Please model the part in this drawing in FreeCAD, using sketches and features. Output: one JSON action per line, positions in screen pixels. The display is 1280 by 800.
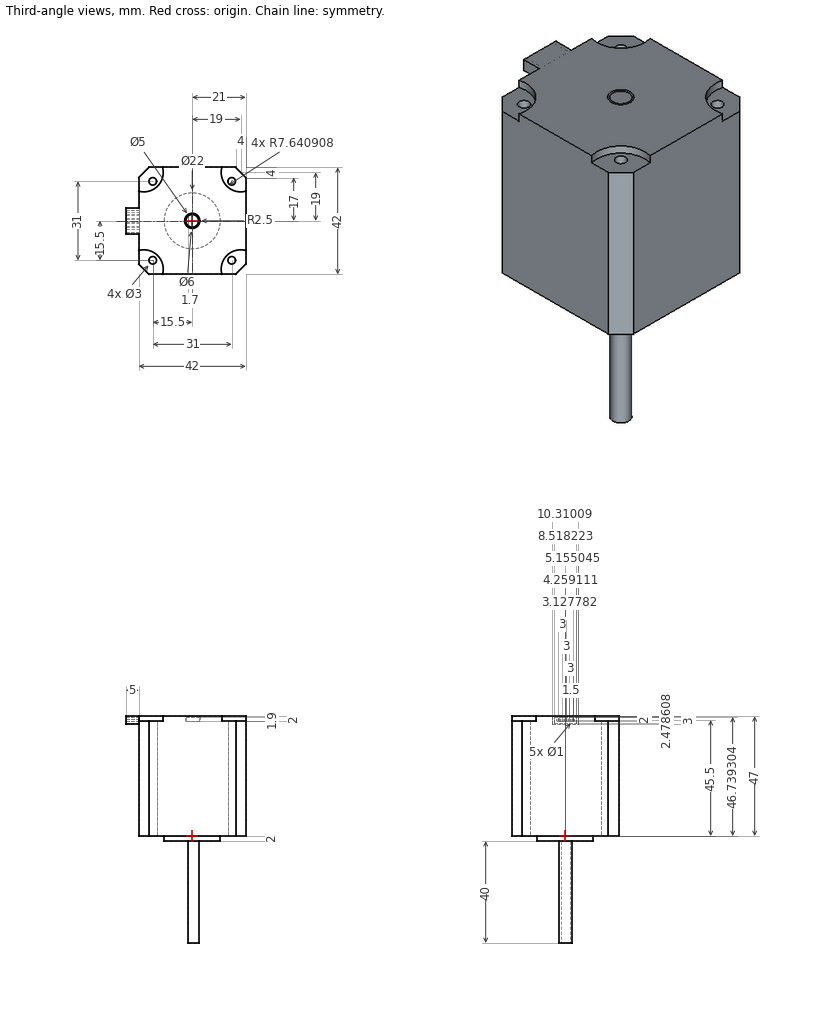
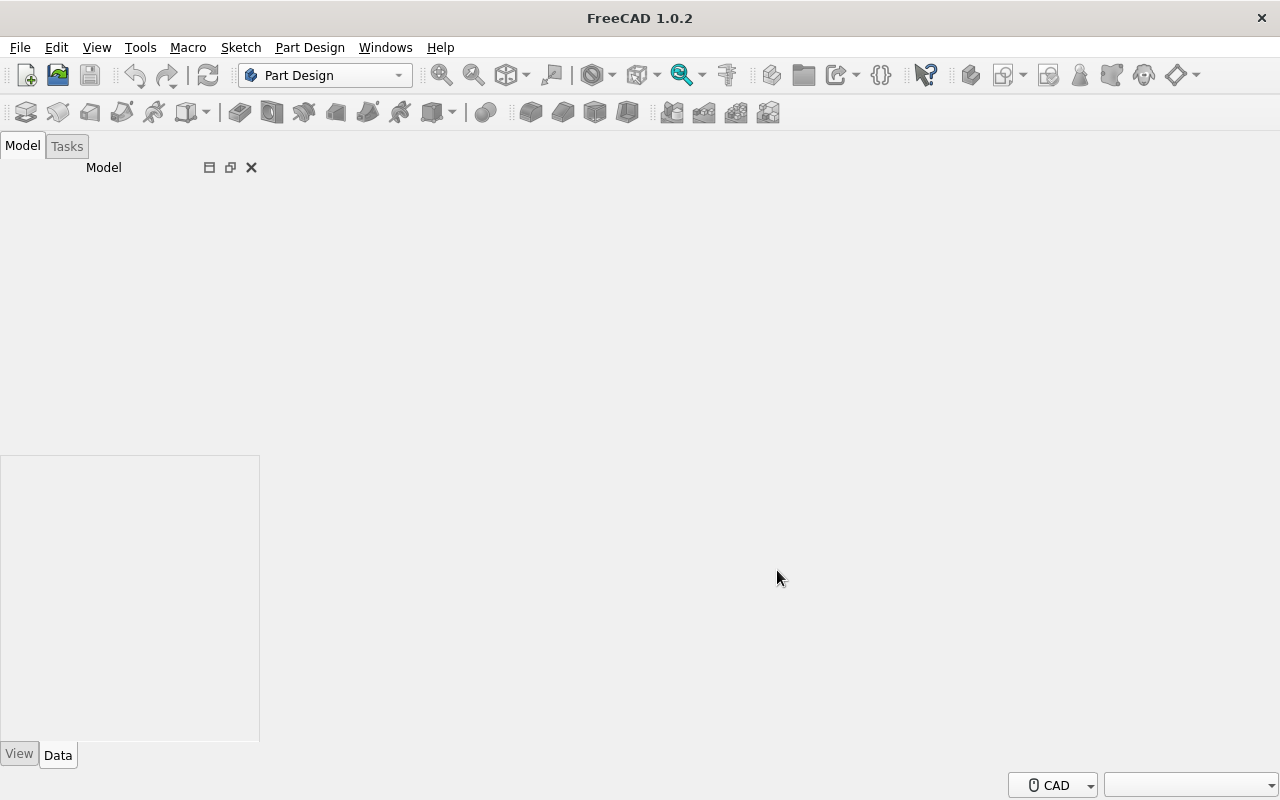
{"action": "left_click", "coordinate": [26, 76]}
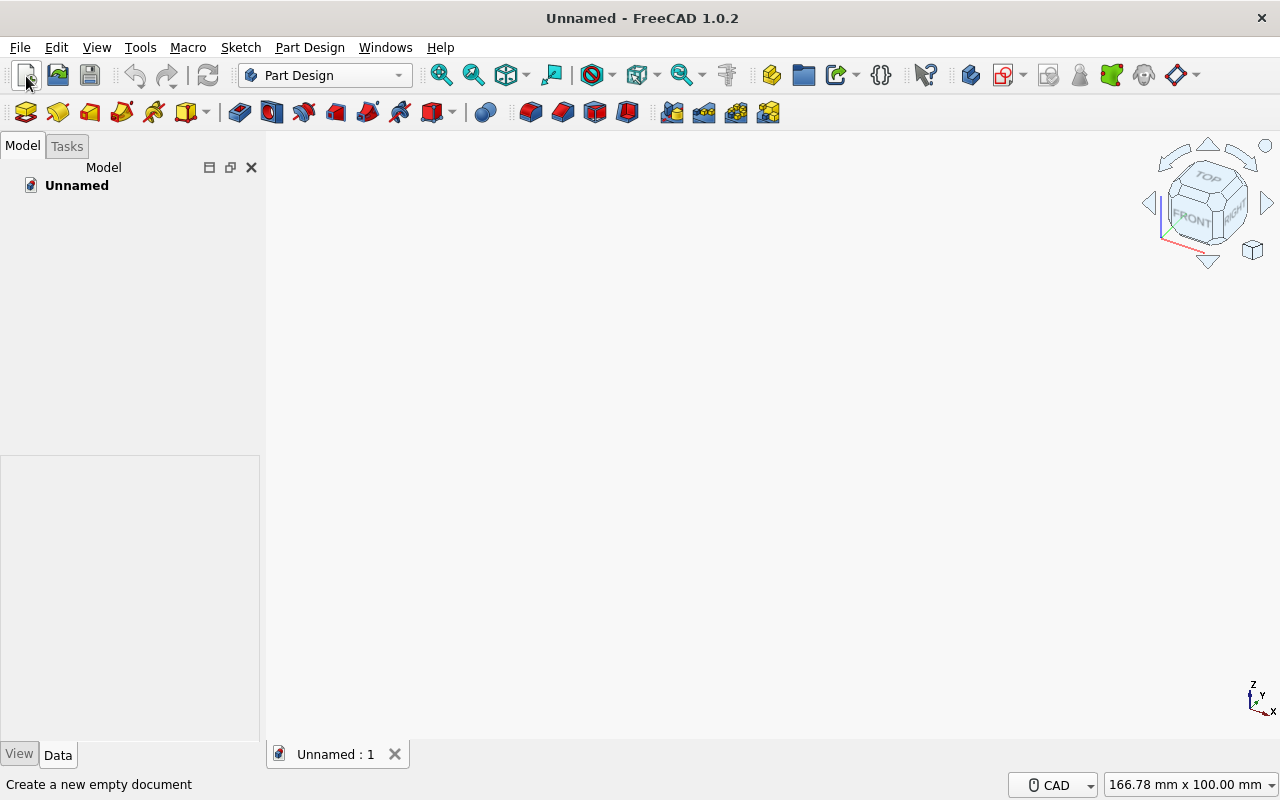
{"action": "left_click", "coordinate": [1004, 76]}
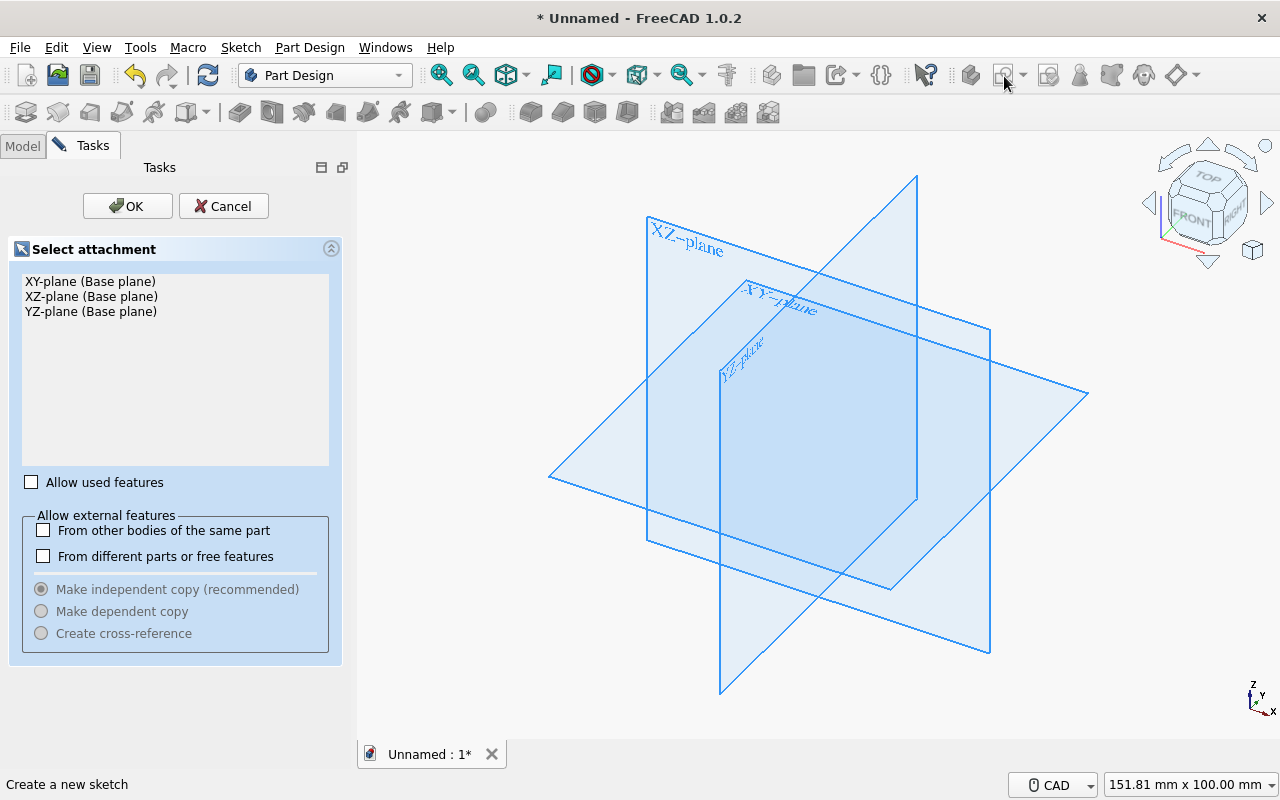
{"action": "left_click", "coordinate": [82, 282]}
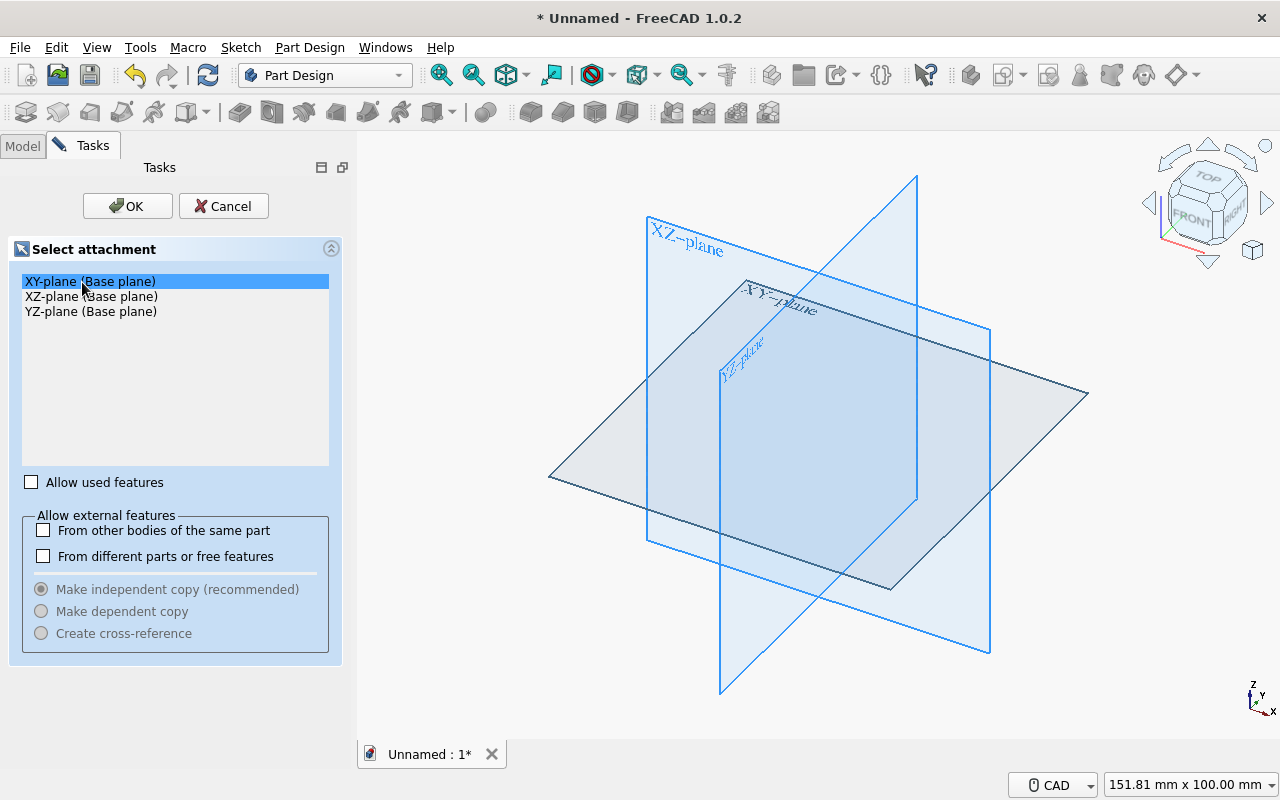
{"action": "left_click", "coordinate": [128, 206]}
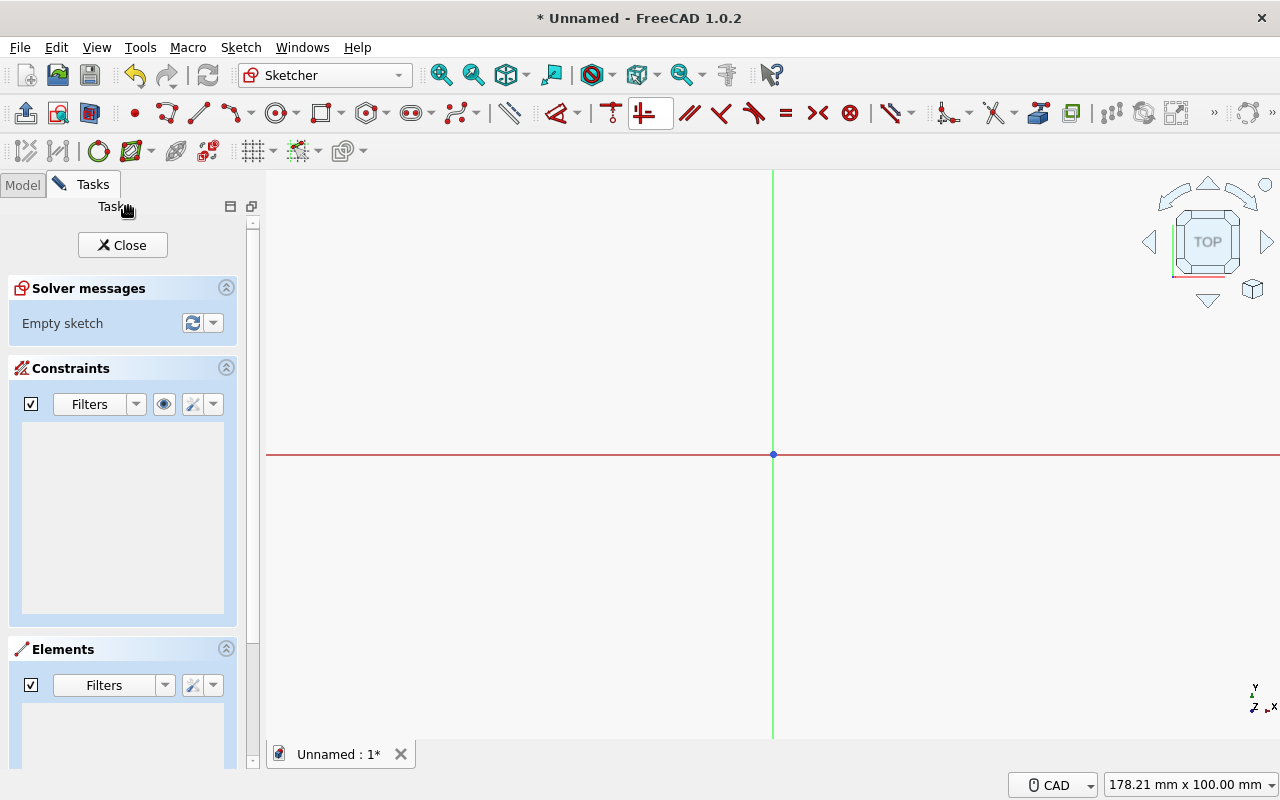
{"action": "scroll", "coordinate": [912, 455], "scroll_direction": "up", "scroll_amount": 2}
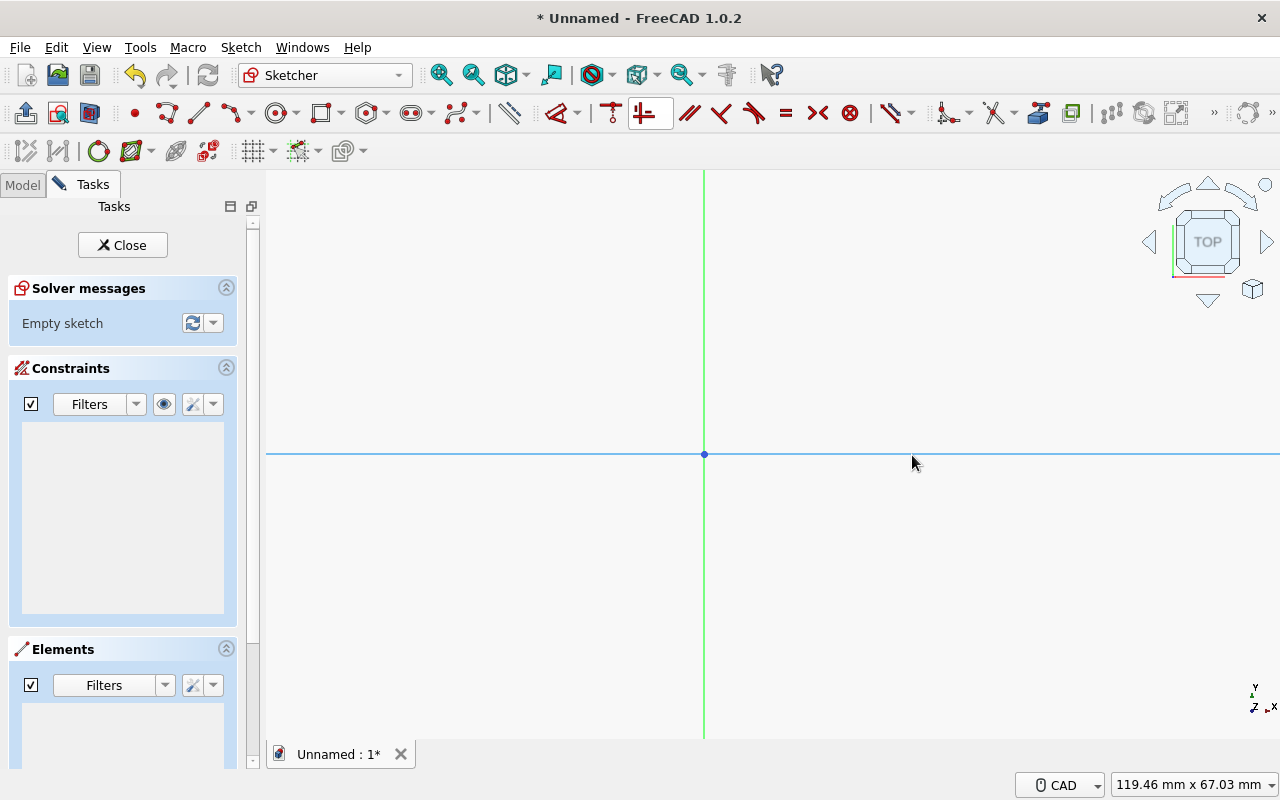
{"action": "left_click", "coordinate": [344, 114]}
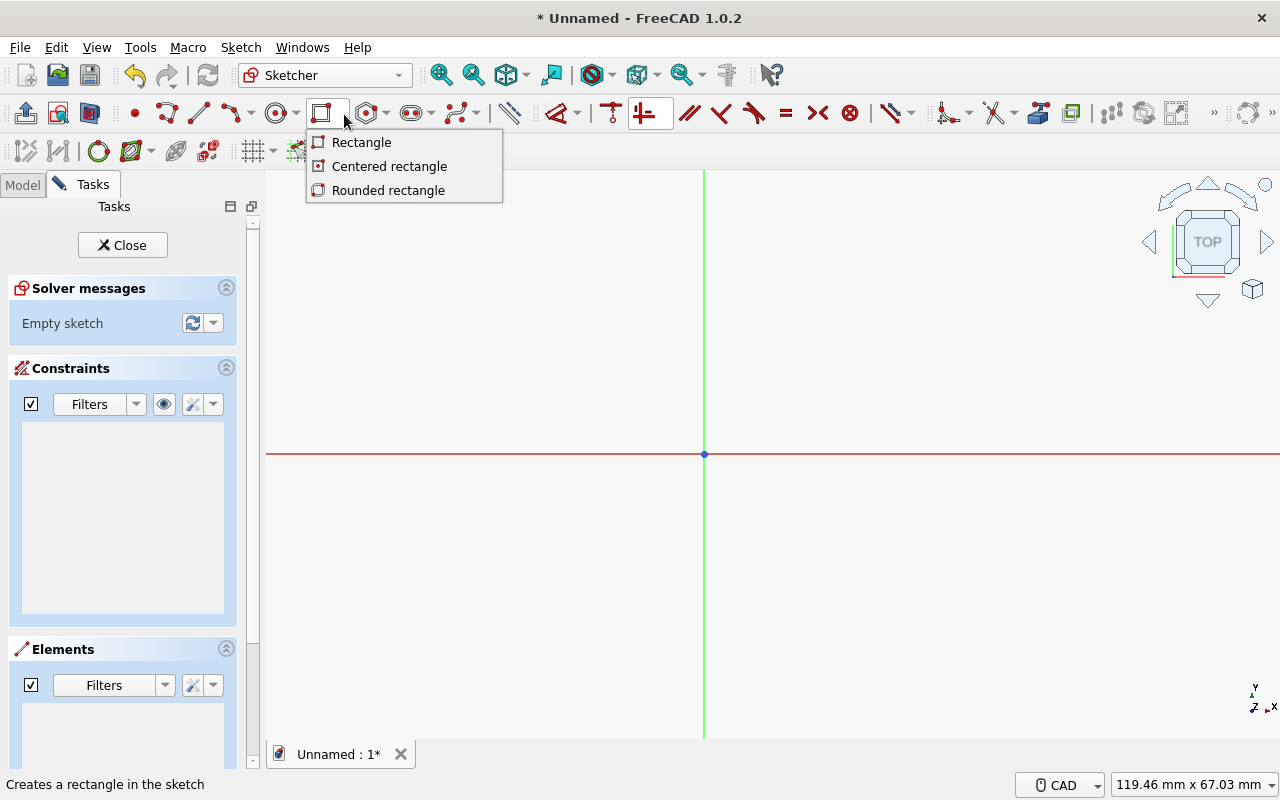
{"action": "left_click", "coordinate": [404, 166]}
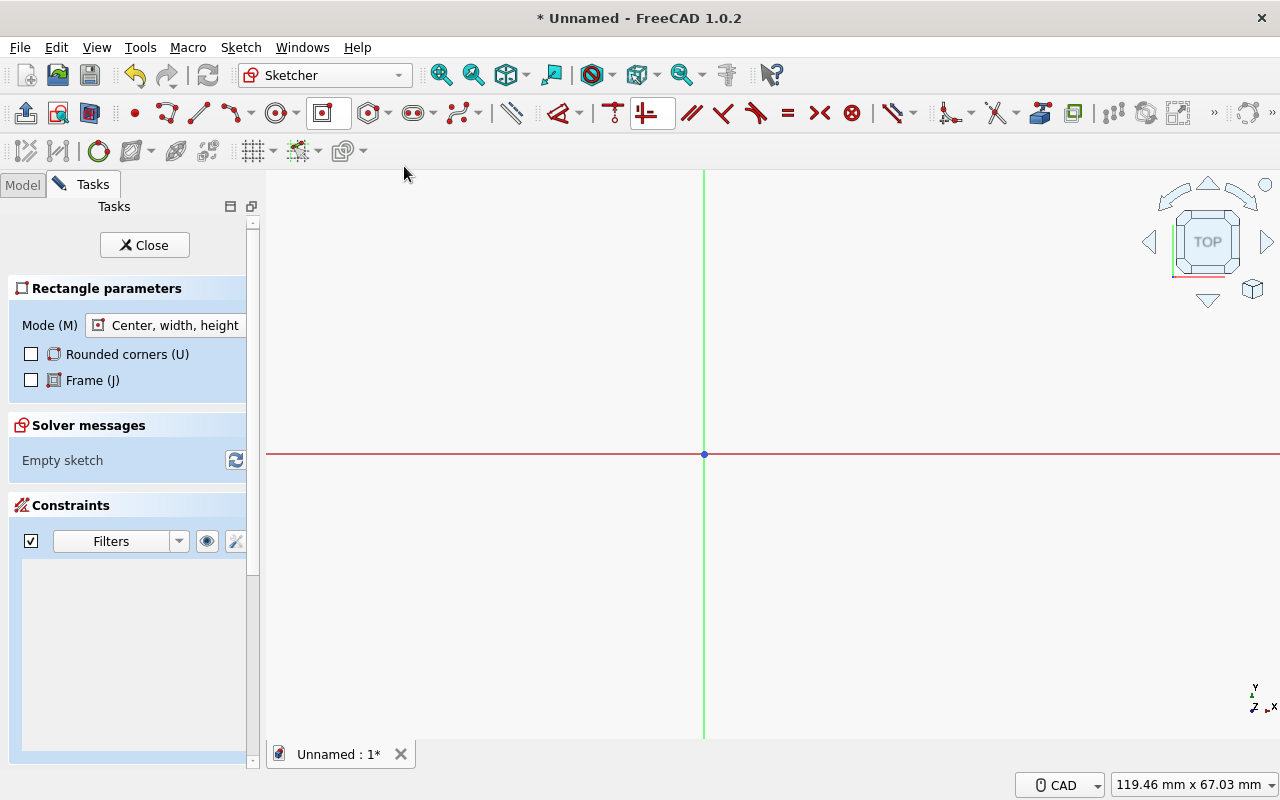
{"action": "left_click", "coordinate": [704, 454]}
{"action": "left_click", "coordinate": [883, 276]}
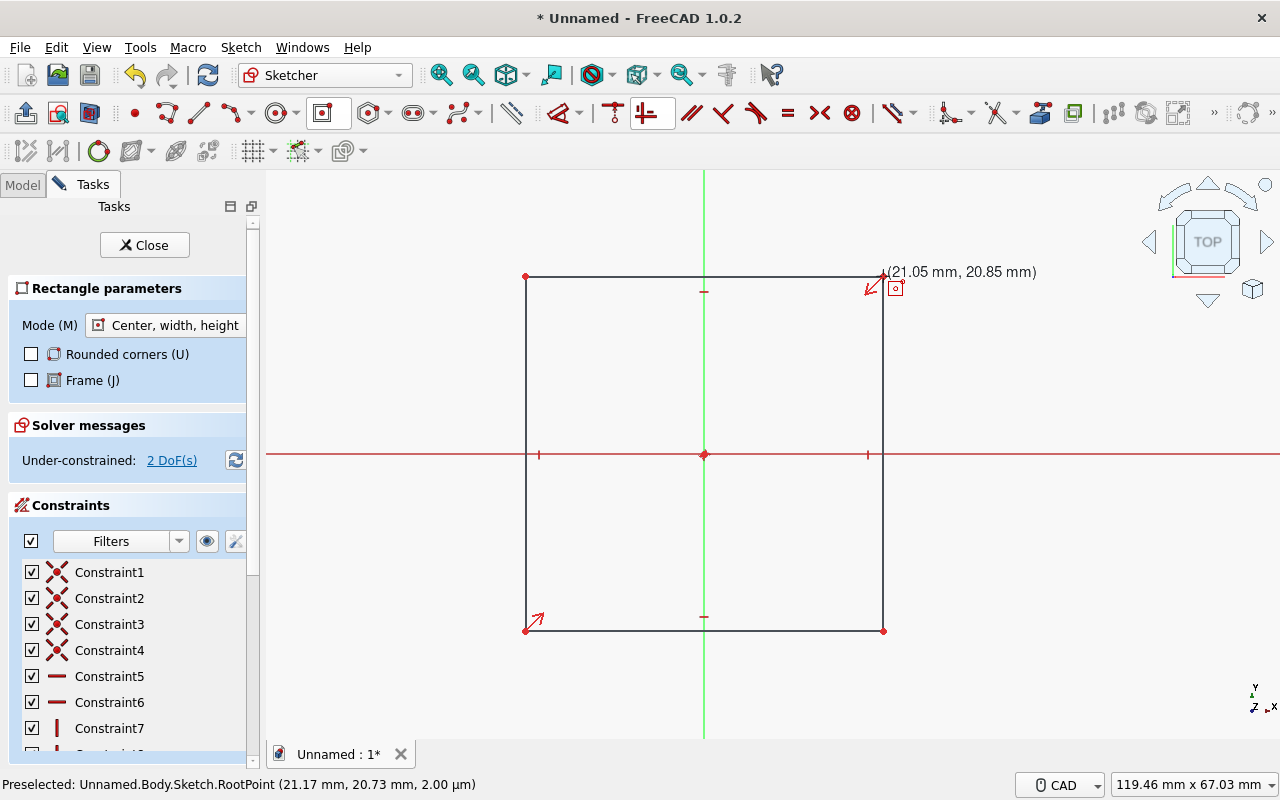
{"action": "left_click", "coordinate": [276, 114]}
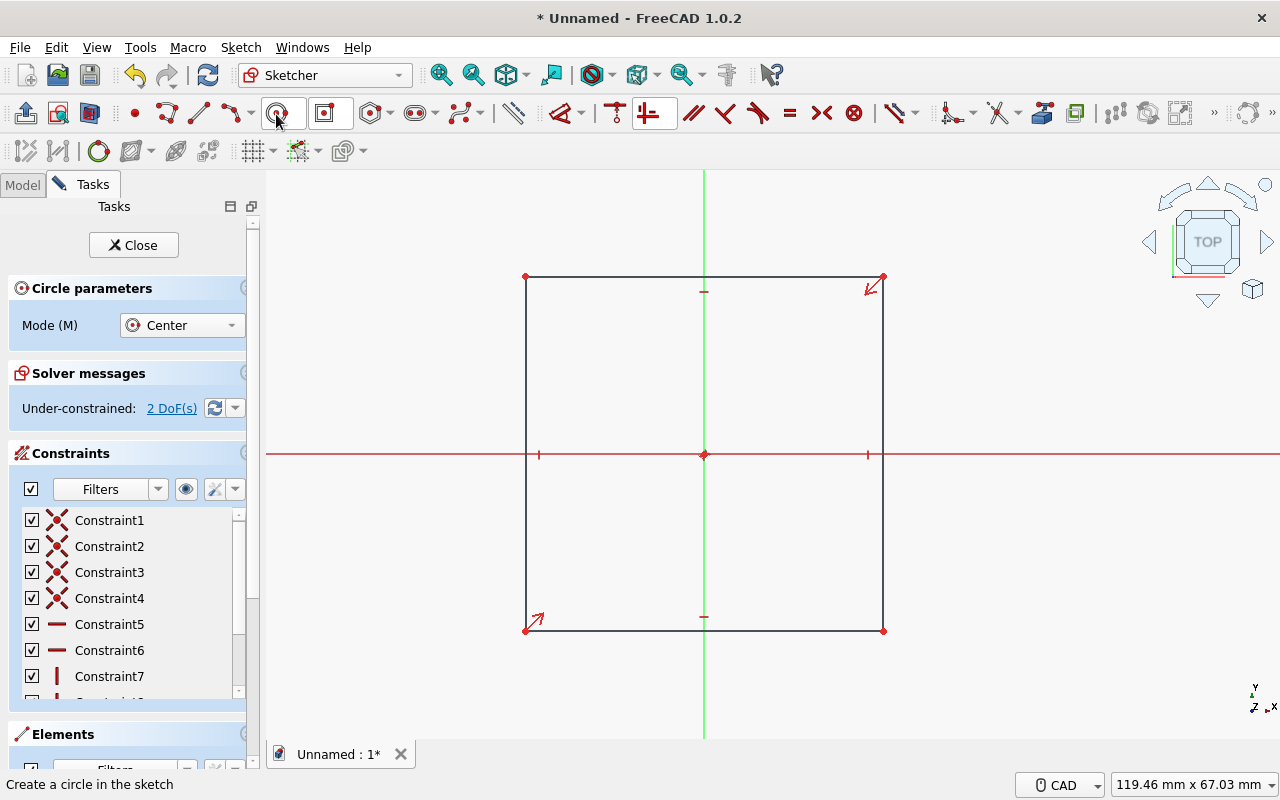
{"action": "scroll", "coordinate": [573, 586], "scroll_direction": "up", "scroll_amount": 3}